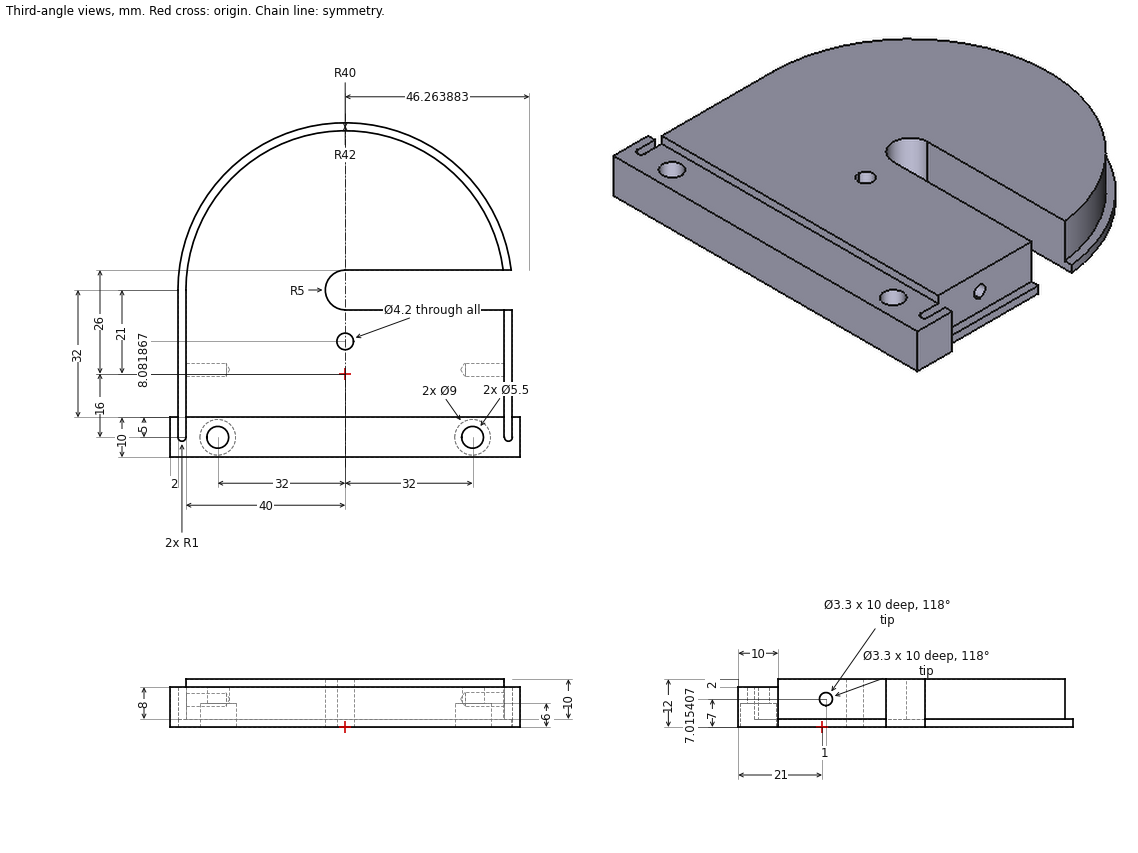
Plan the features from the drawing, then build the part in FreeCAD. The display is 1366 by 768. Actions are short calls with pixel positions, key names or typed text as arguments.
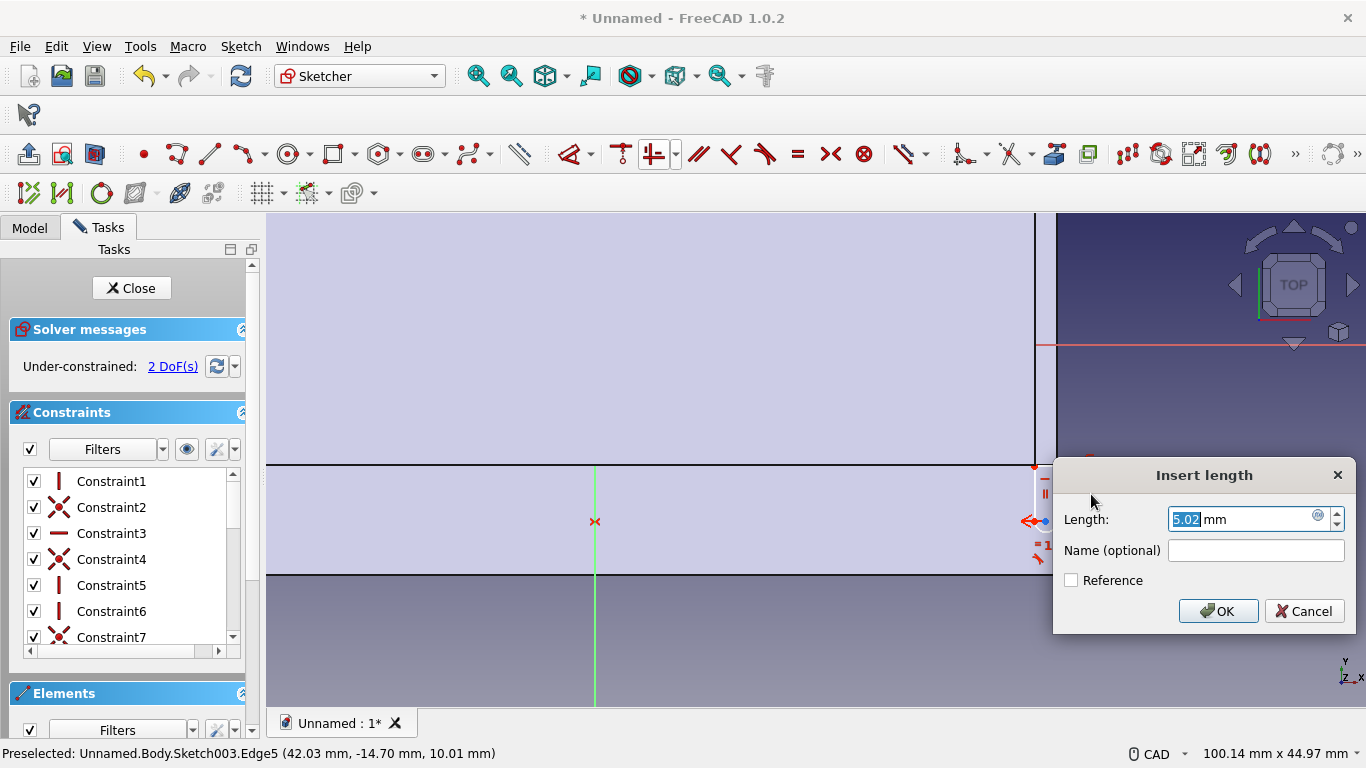
text(5)
key(Return)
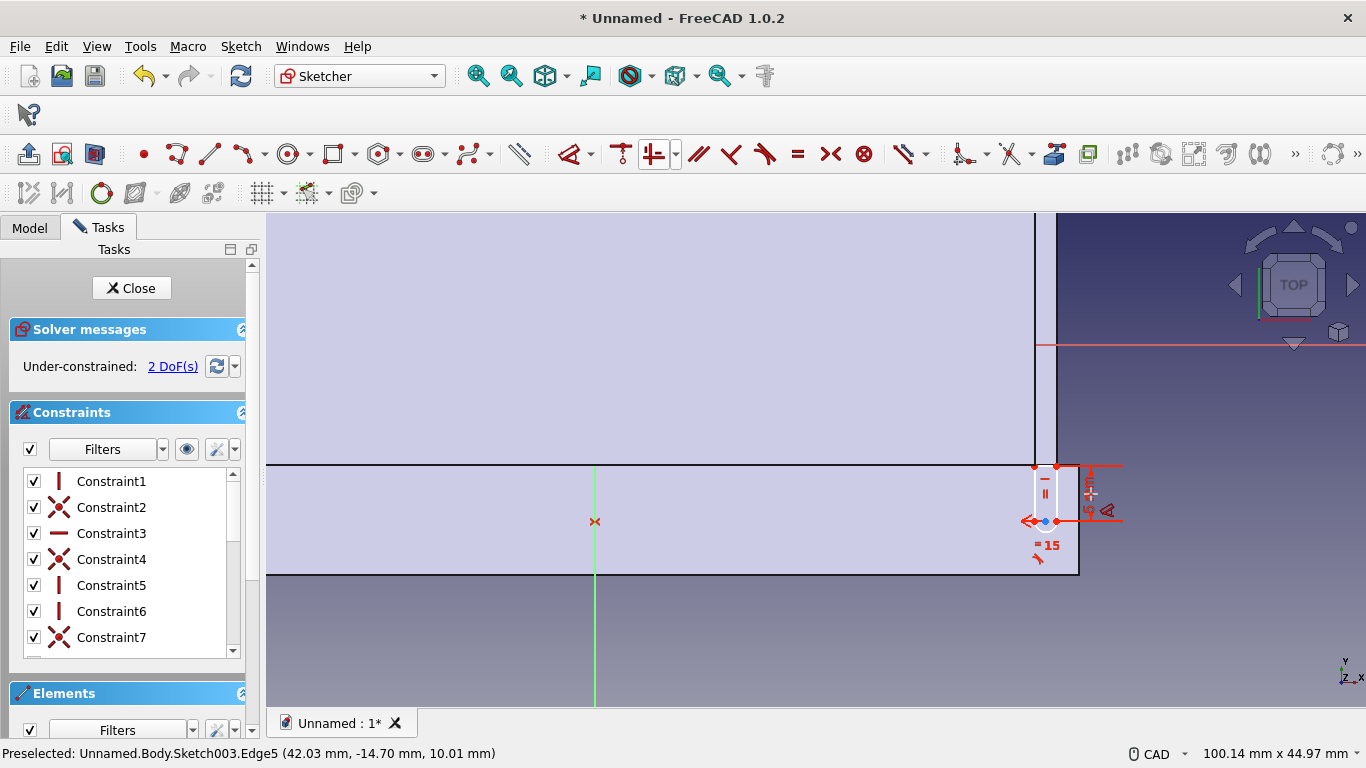
scroll(1057, 505, down, 2)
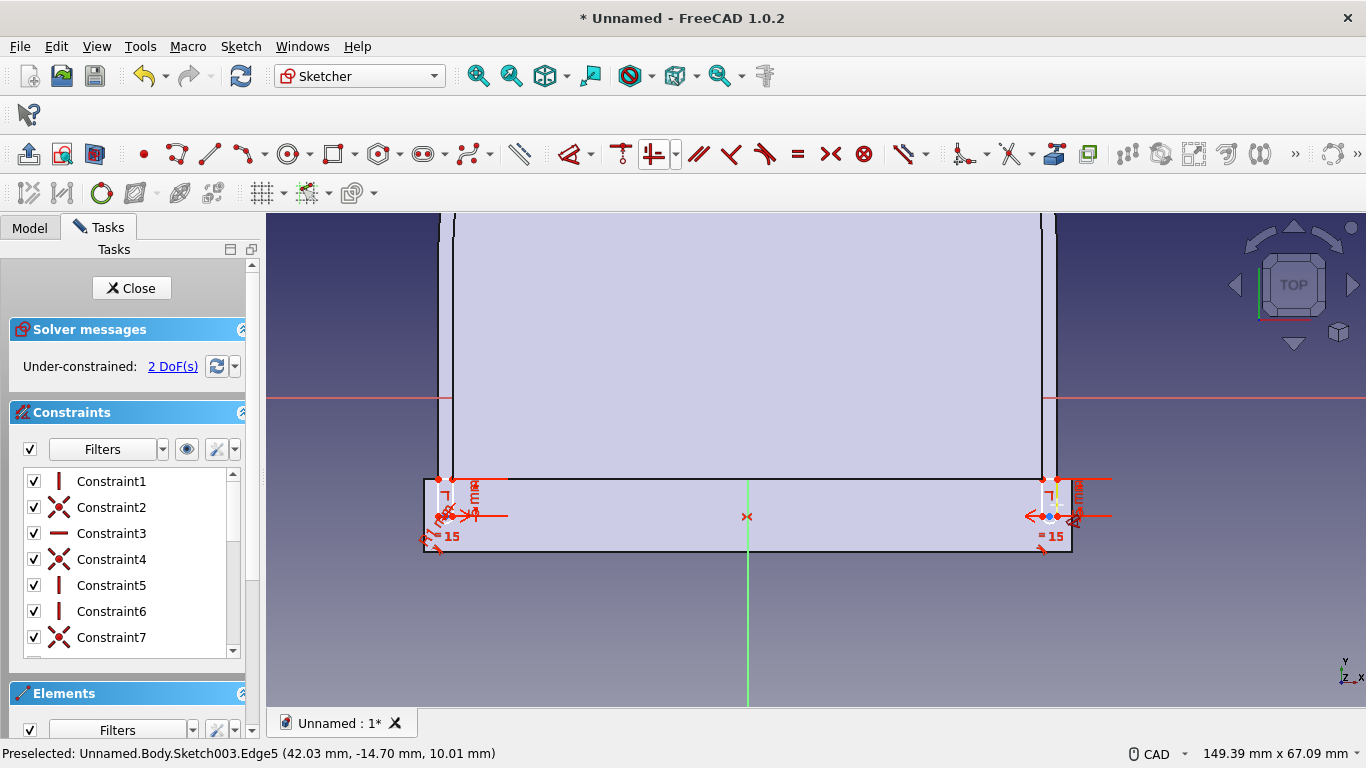
scroll(453, 516, up, 3)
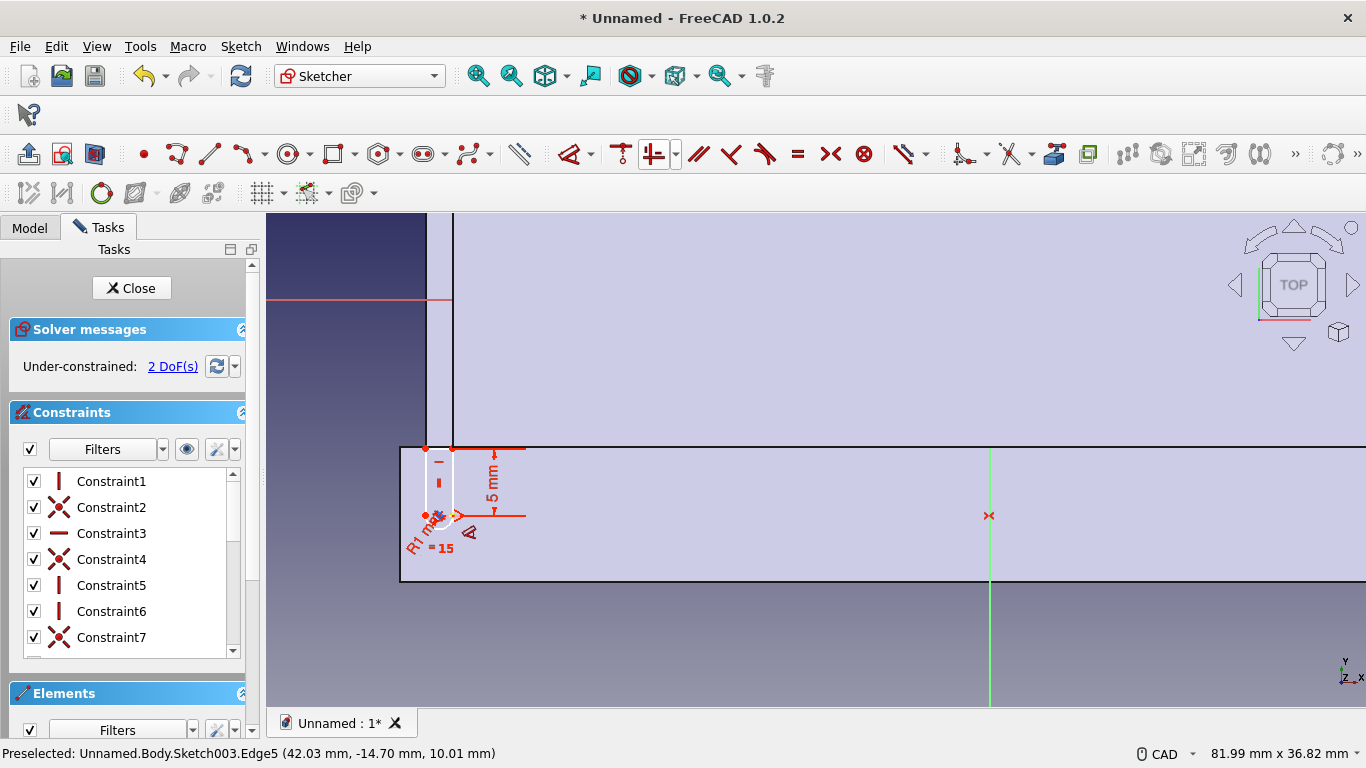
click(453, 516)
click(721, 266)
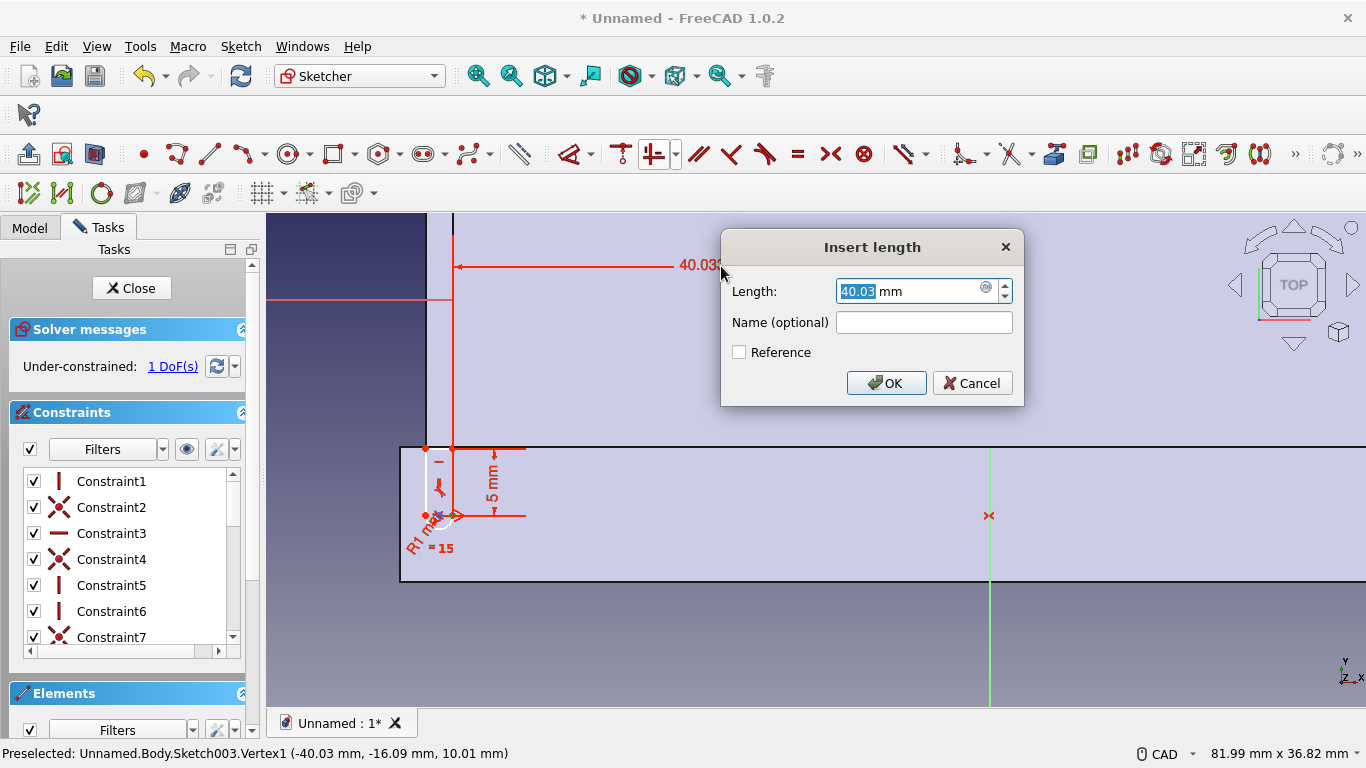
text(40)
key(Return)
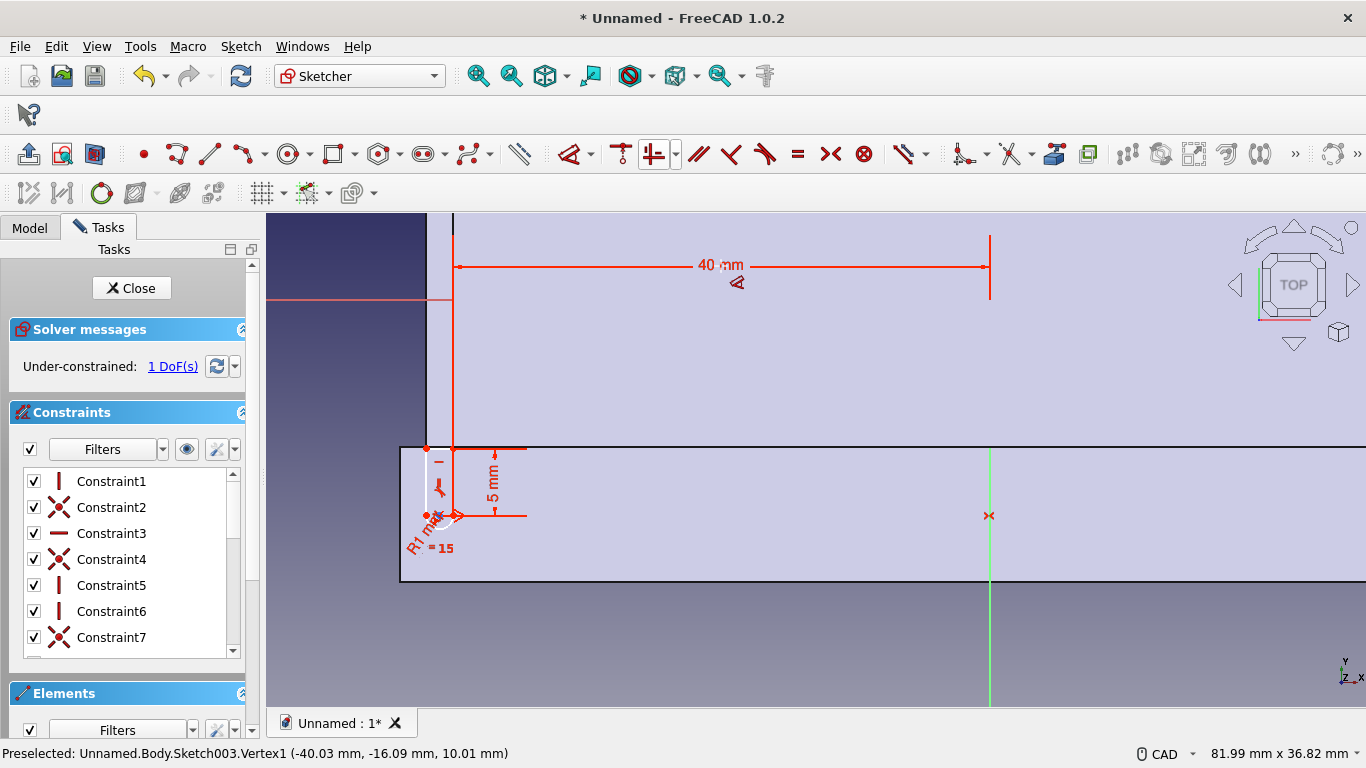
click(453, 516)
click(419, 408)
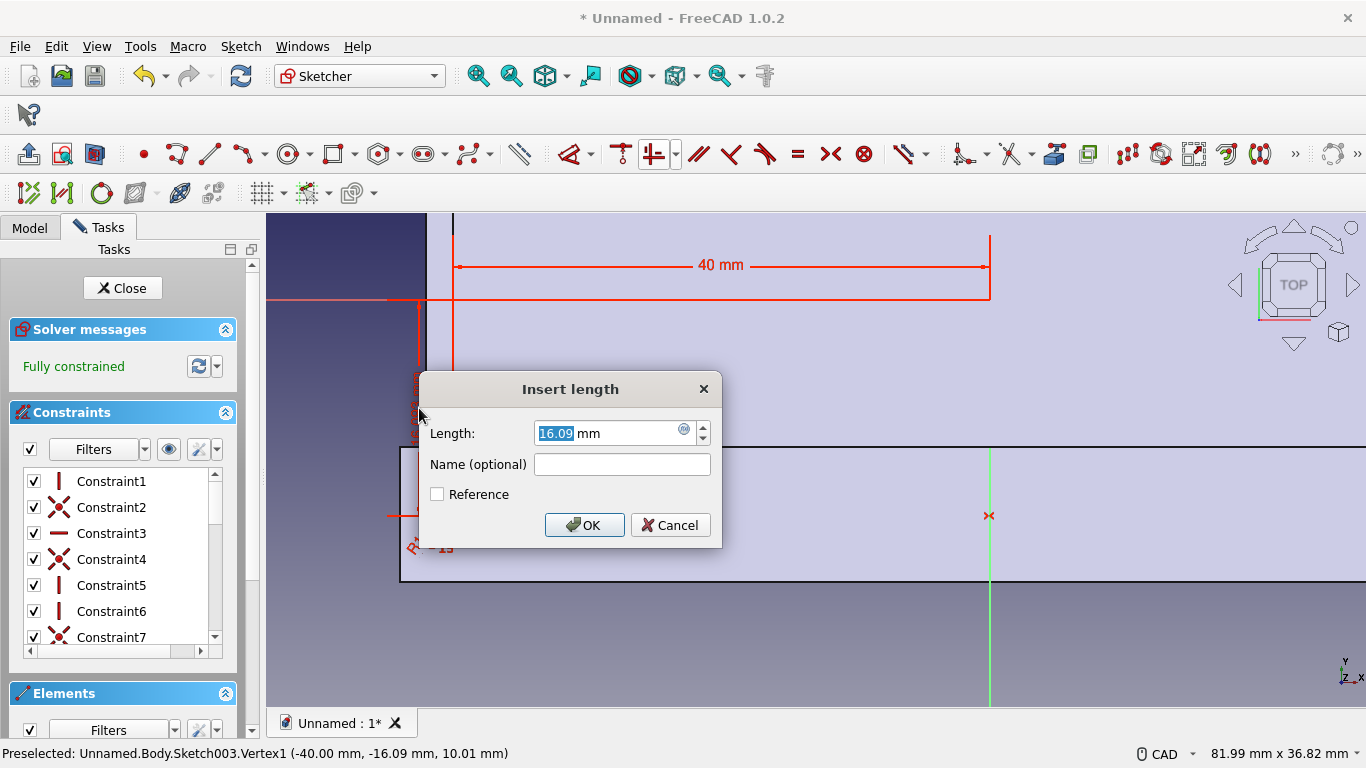
text(16)
key(Return)
key(Escape)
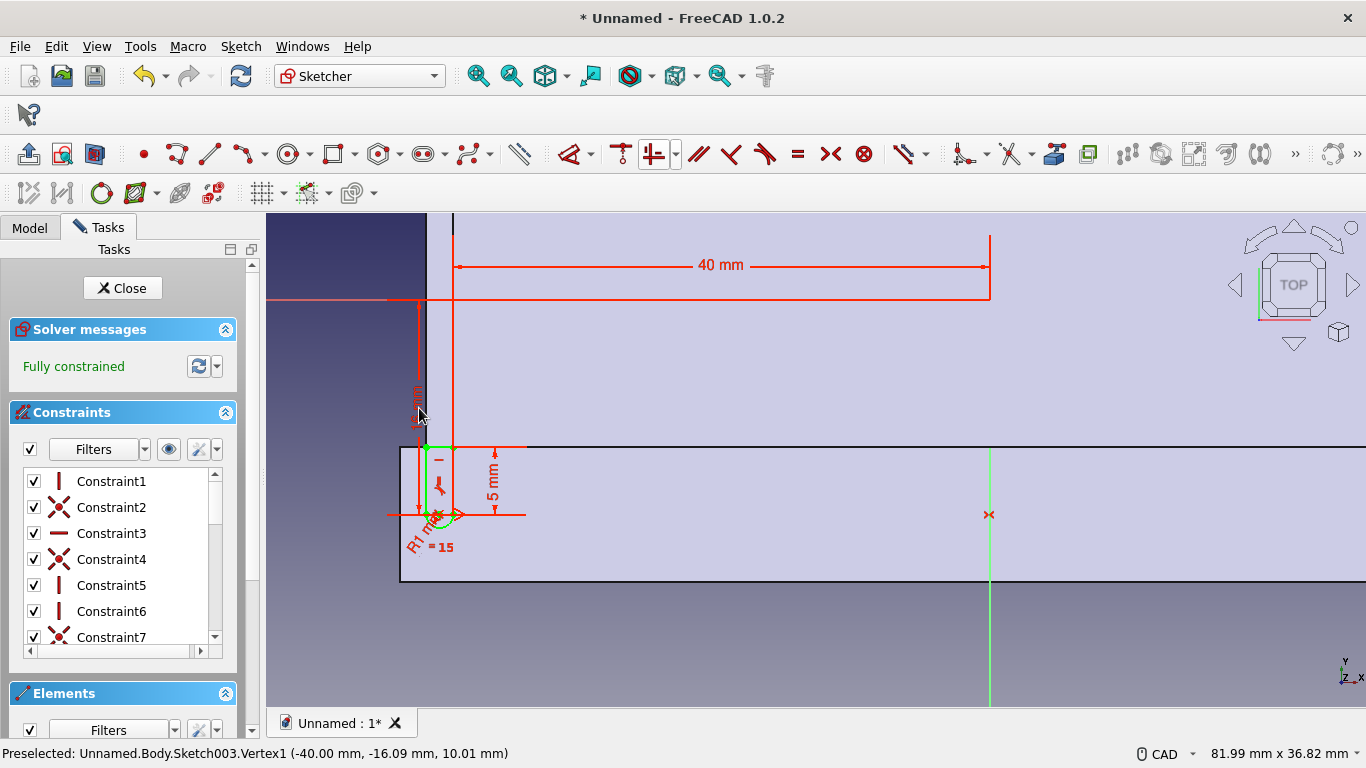
click(123, 288)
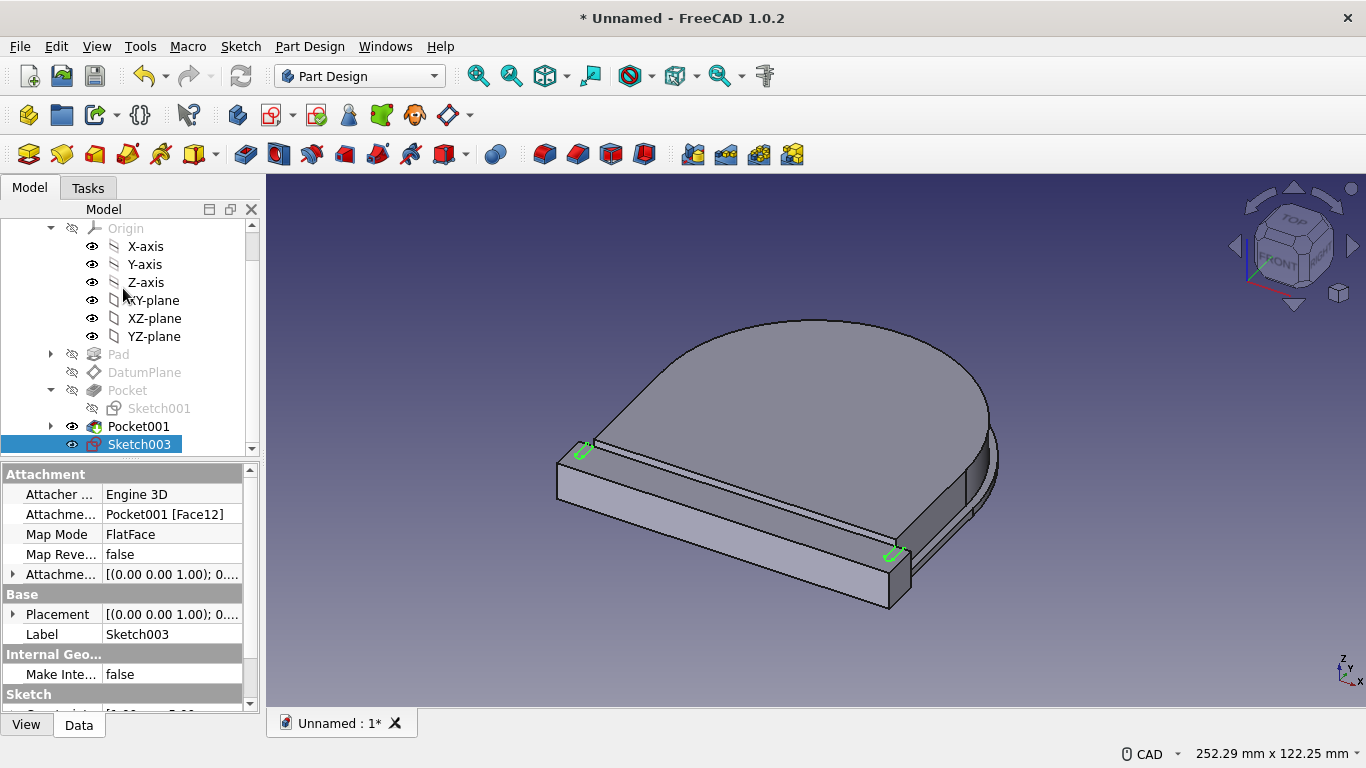
click(246, 154)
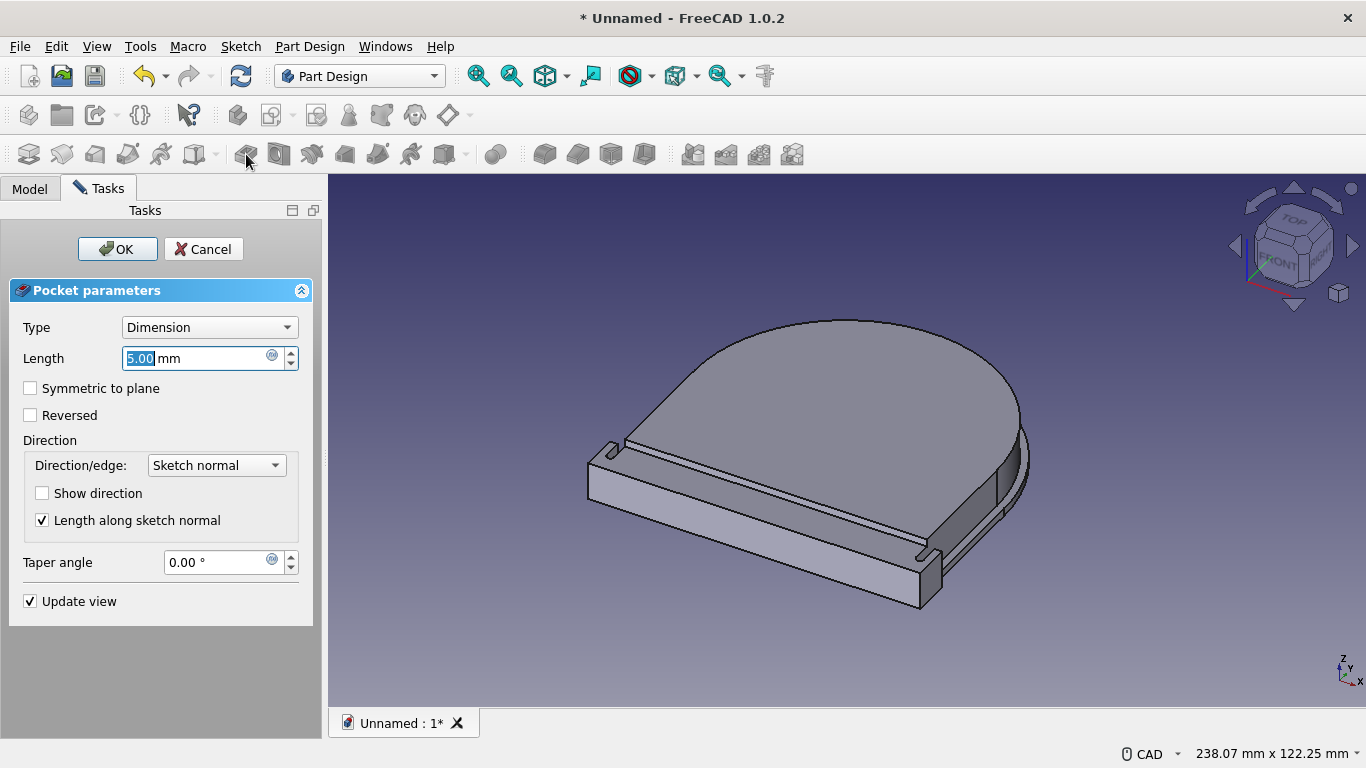
text(8)
key(Tab)